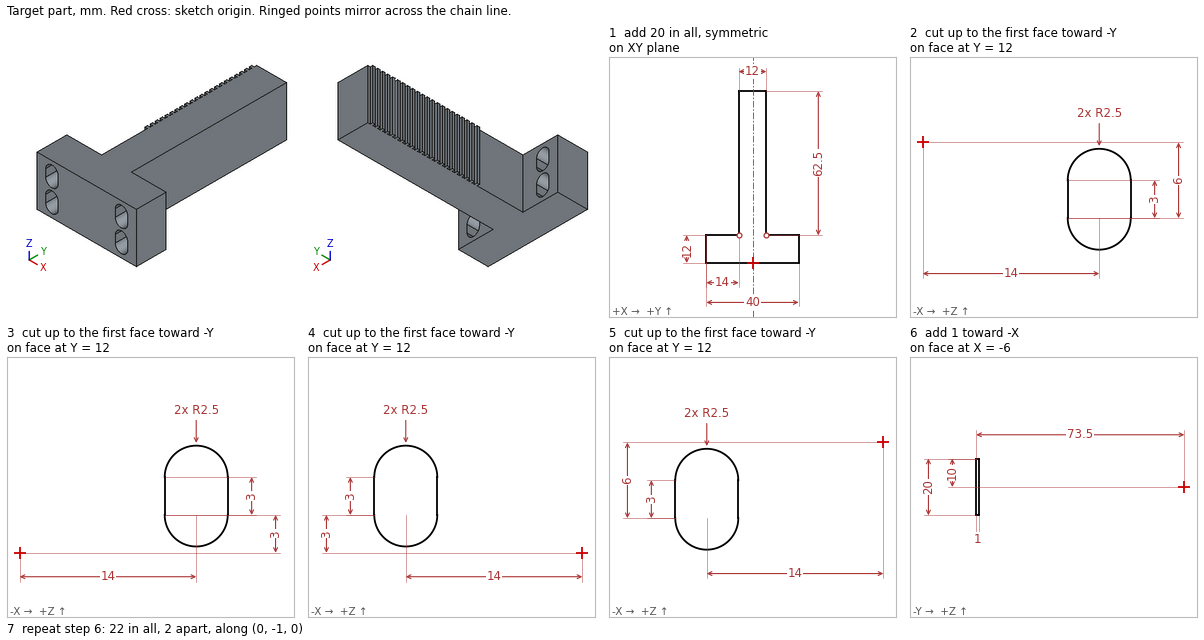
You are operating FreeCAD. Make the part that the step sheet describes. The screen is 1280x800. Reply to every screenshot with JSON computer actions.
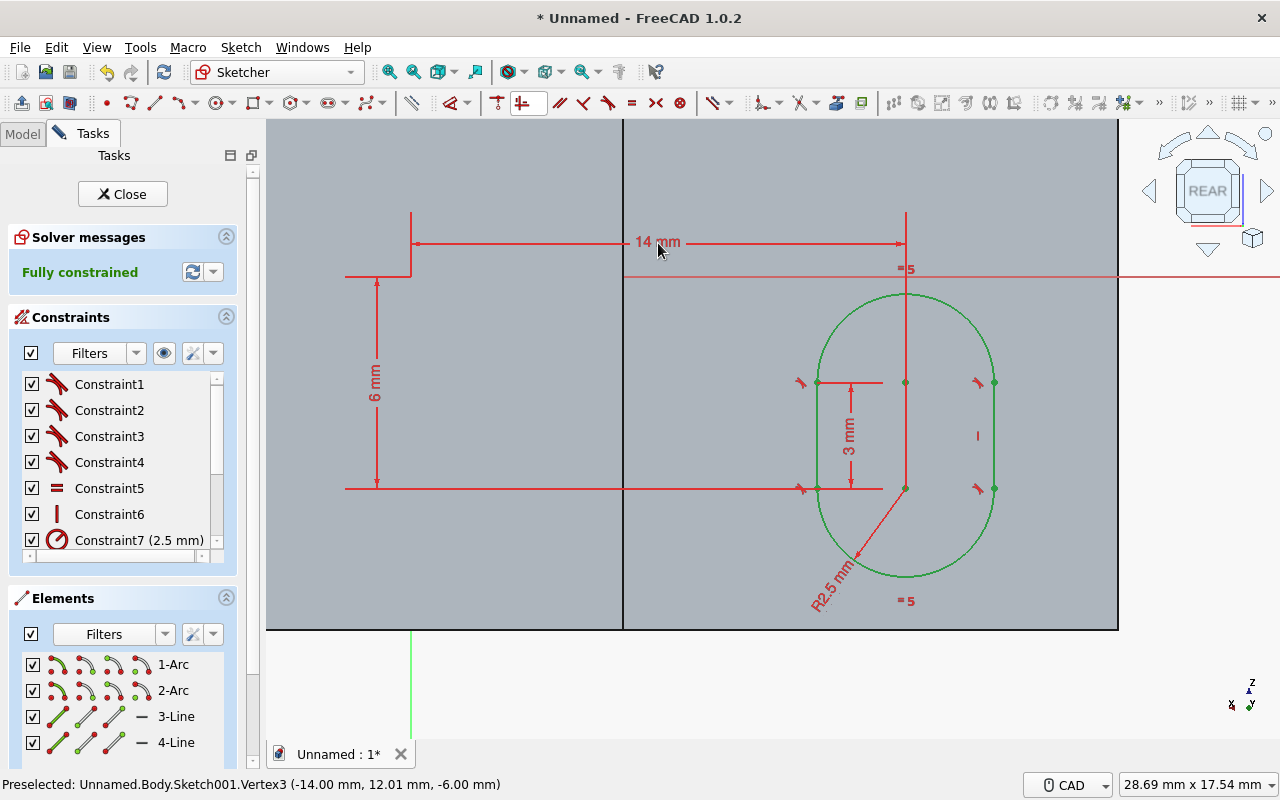
{"action": "left_click", "coordinate": [123, 194]}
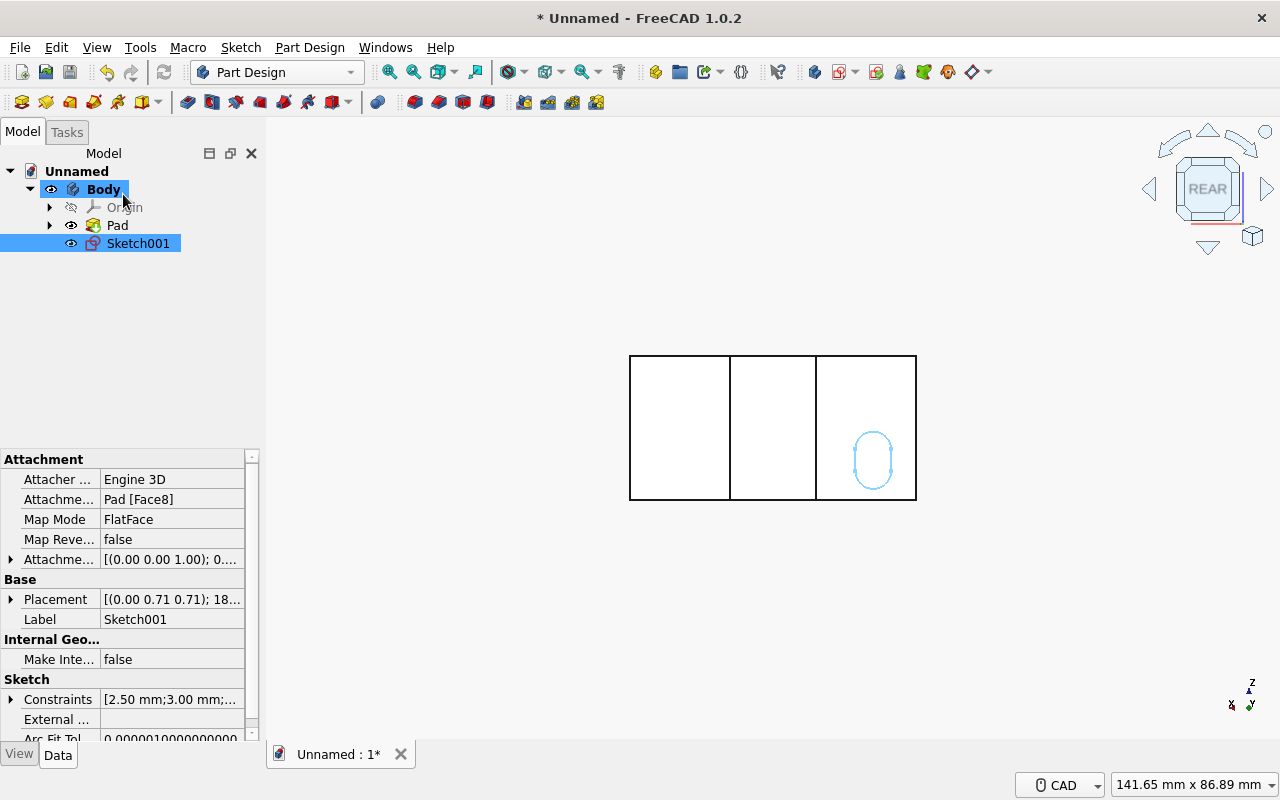
{"action": "left_click", "coordinate": [188, 102]}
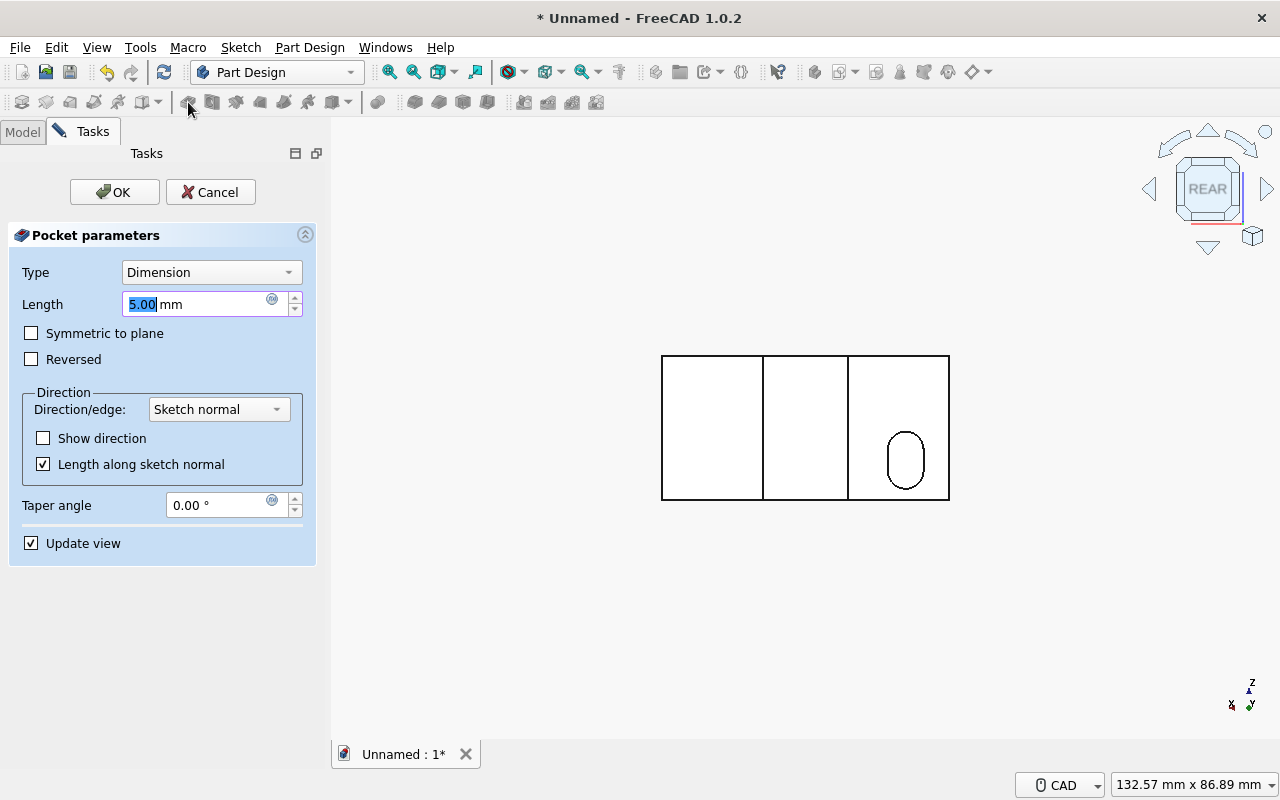
{"action": "left_click", "coordinate": [212, 272]}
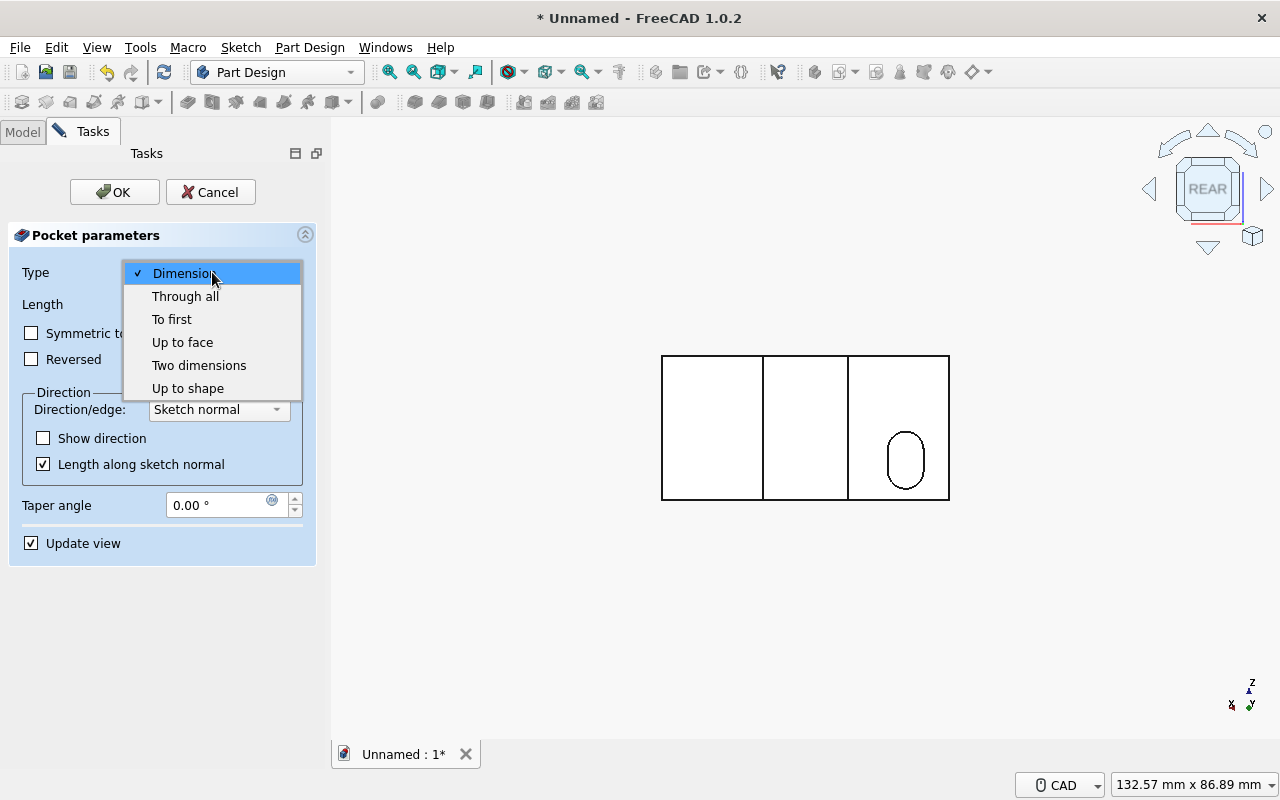
{"action": "left_click", "coordinate": [212, 320]}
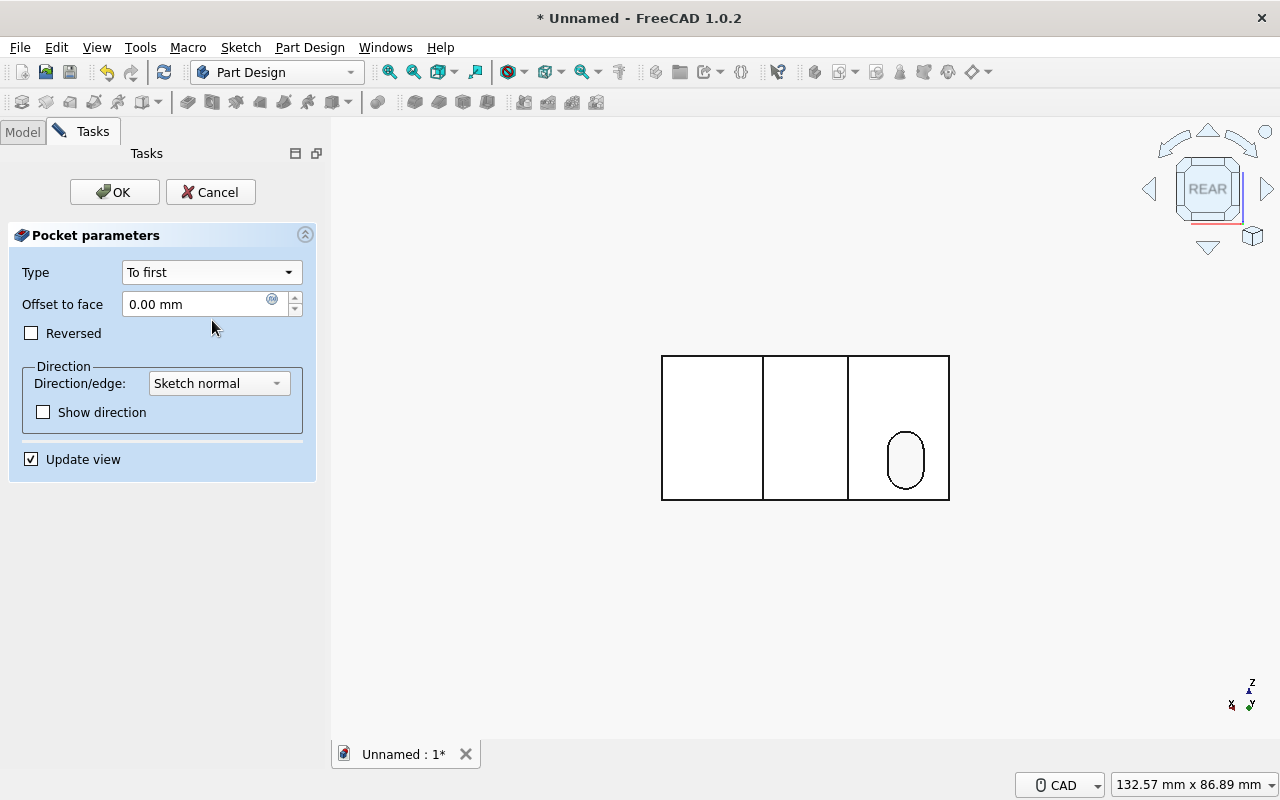
{"action": "left_click", "coordinate": [115, 192]}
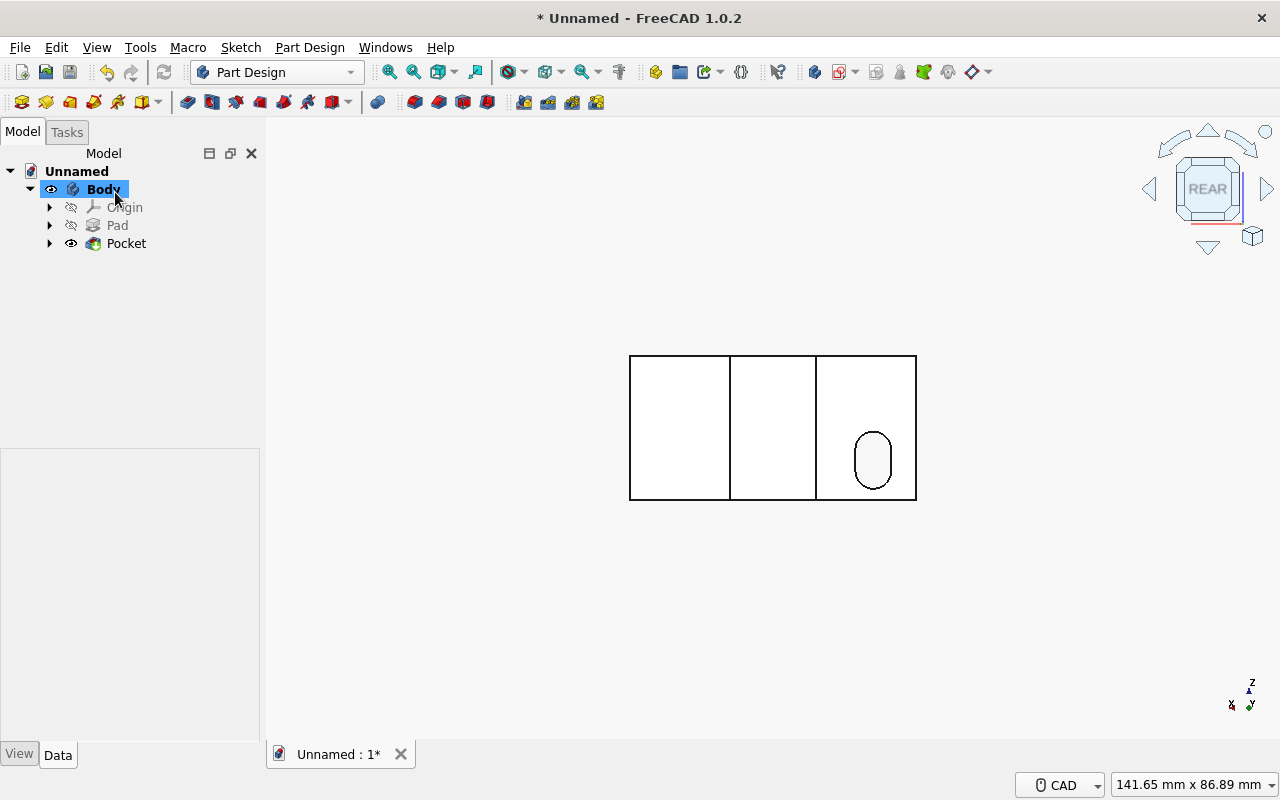
{"action": "key", "text": "v f"}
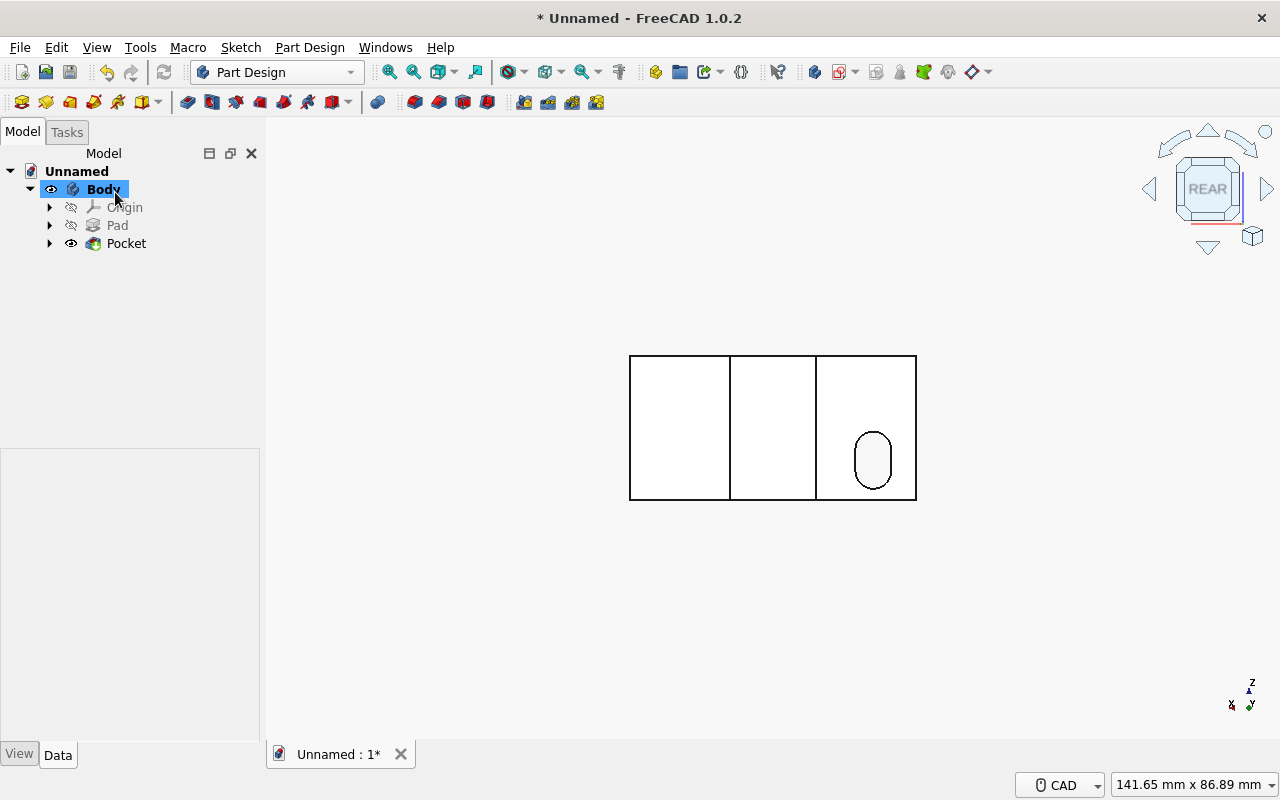
{"action": "left_click", "coordinate": [680, 407]}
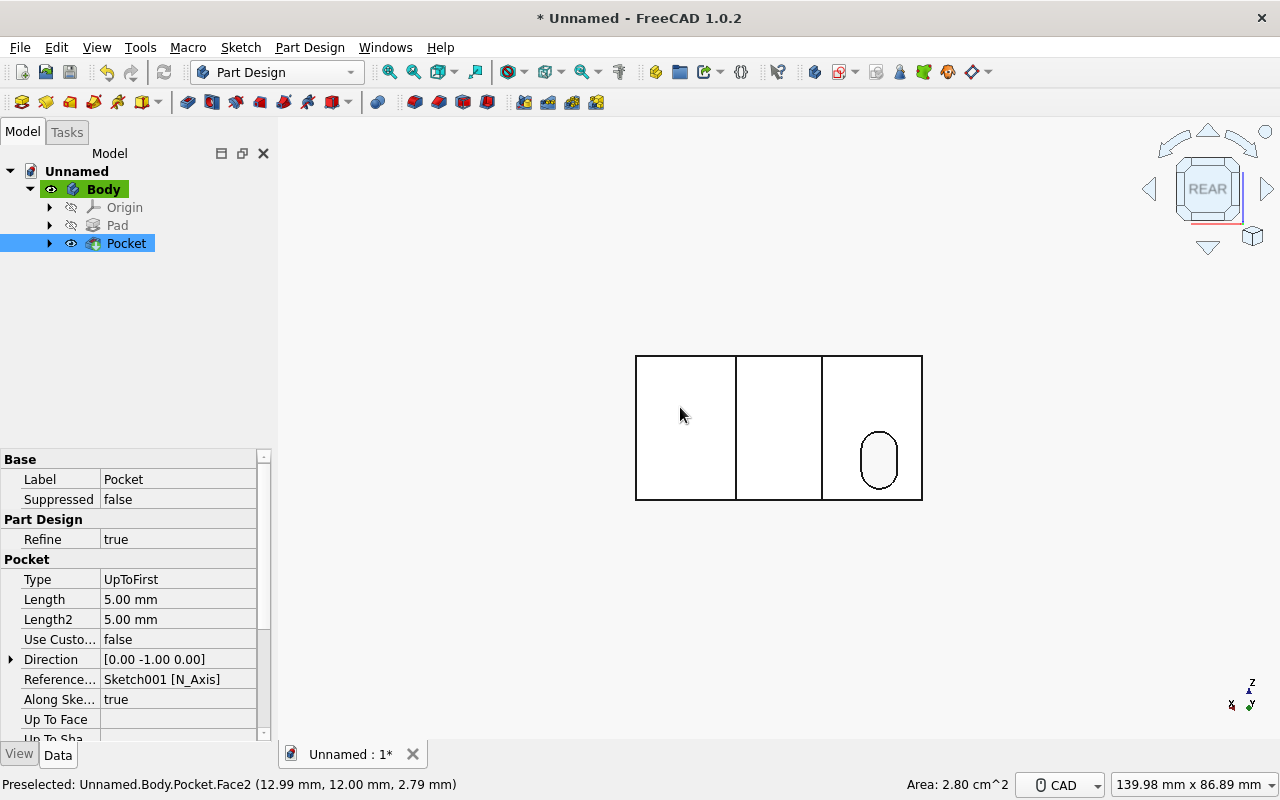
{"action": "left_click", "coordinate": [840, 72]}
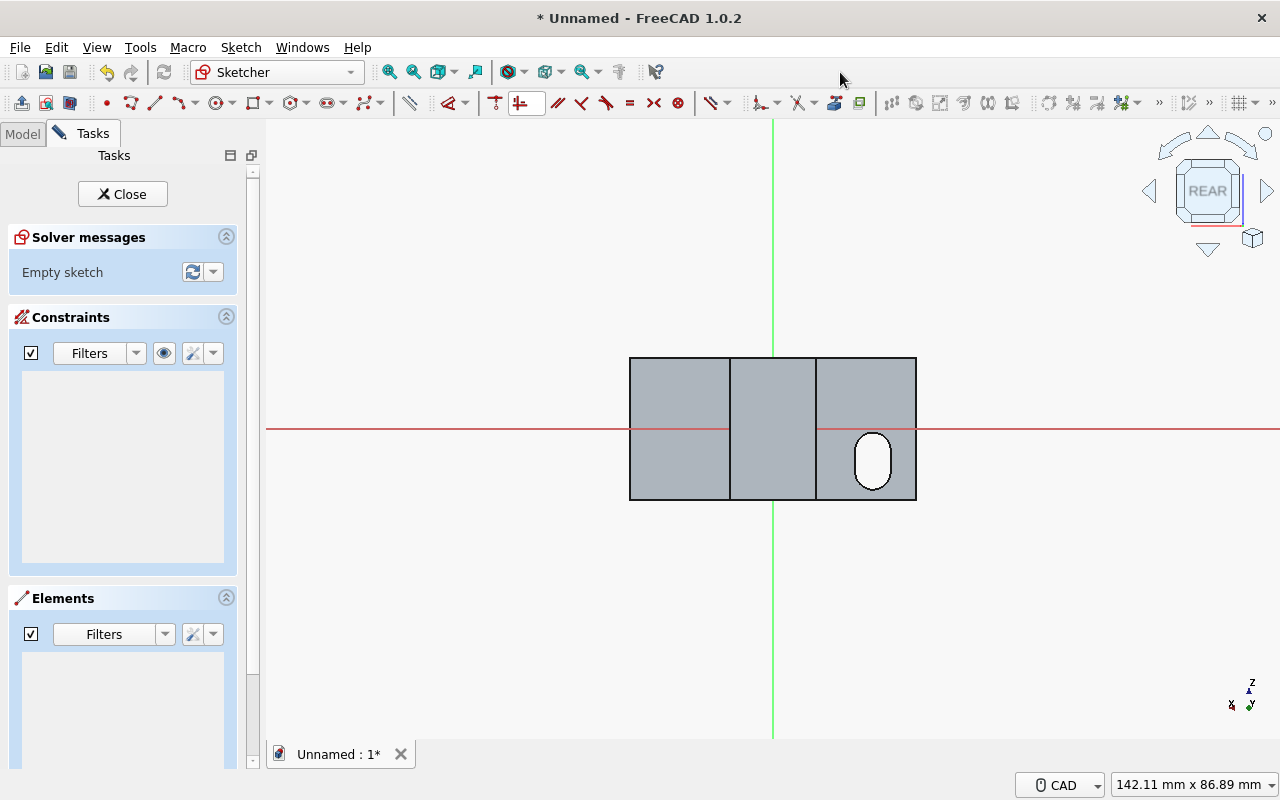
{"action": "left_click", "coordinate": [70, 104]}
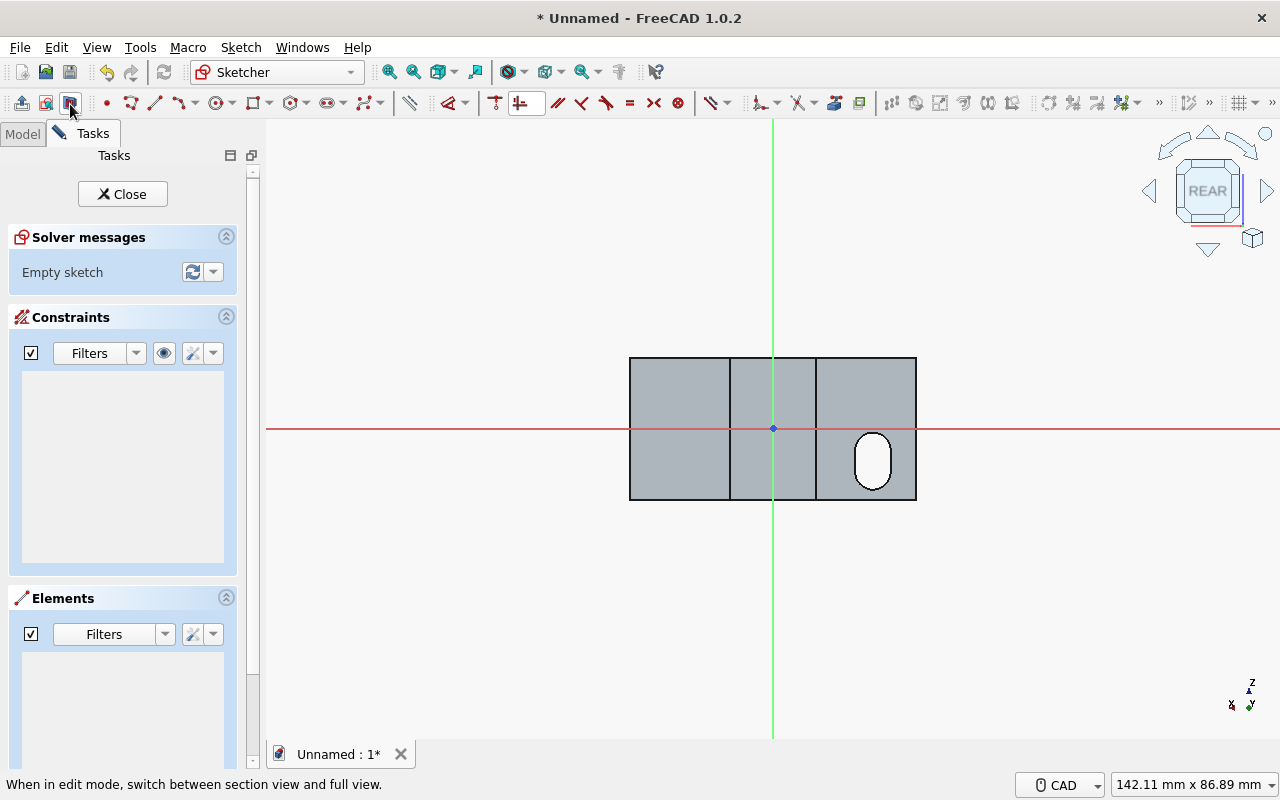
{"action": "scroll", "coordinate": [864, 391], "scroll_direction": "up", "scroll_amount": 8}